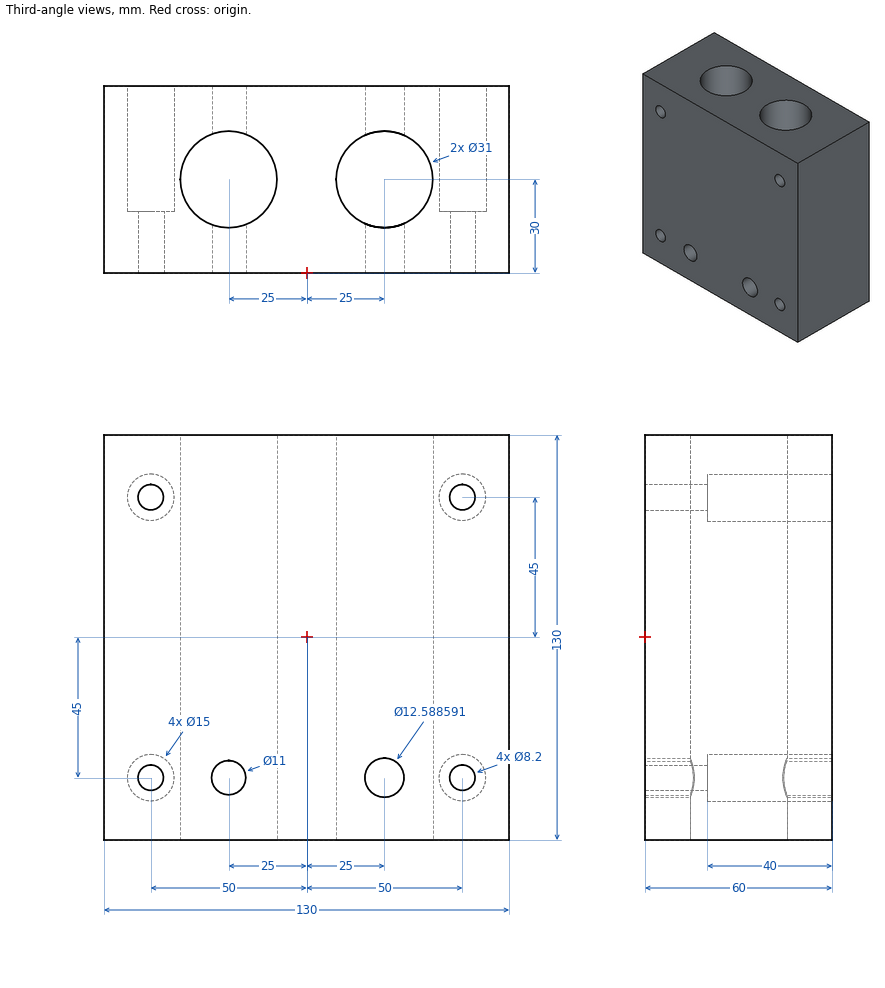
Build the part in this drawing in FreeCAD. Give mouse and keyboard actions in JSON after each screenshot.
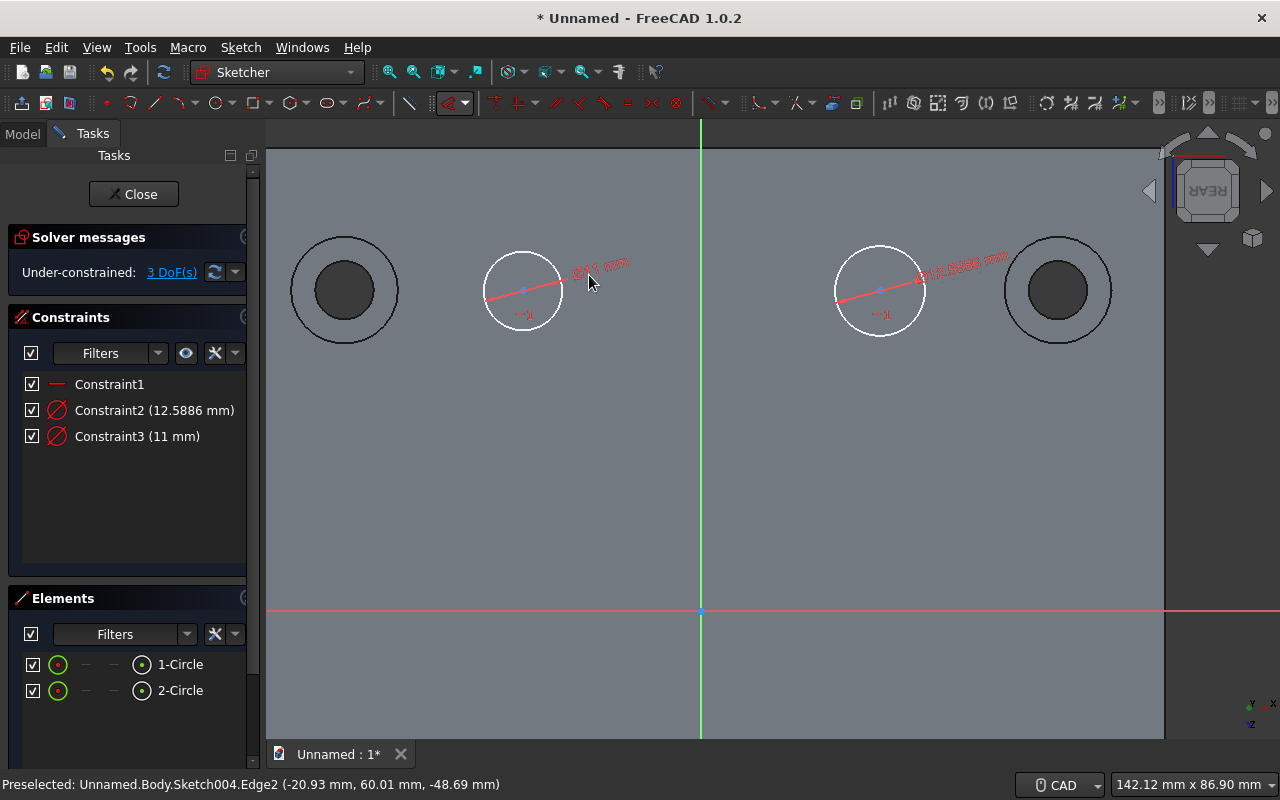
{"action": "left_click", "coordinate": [880, 291]}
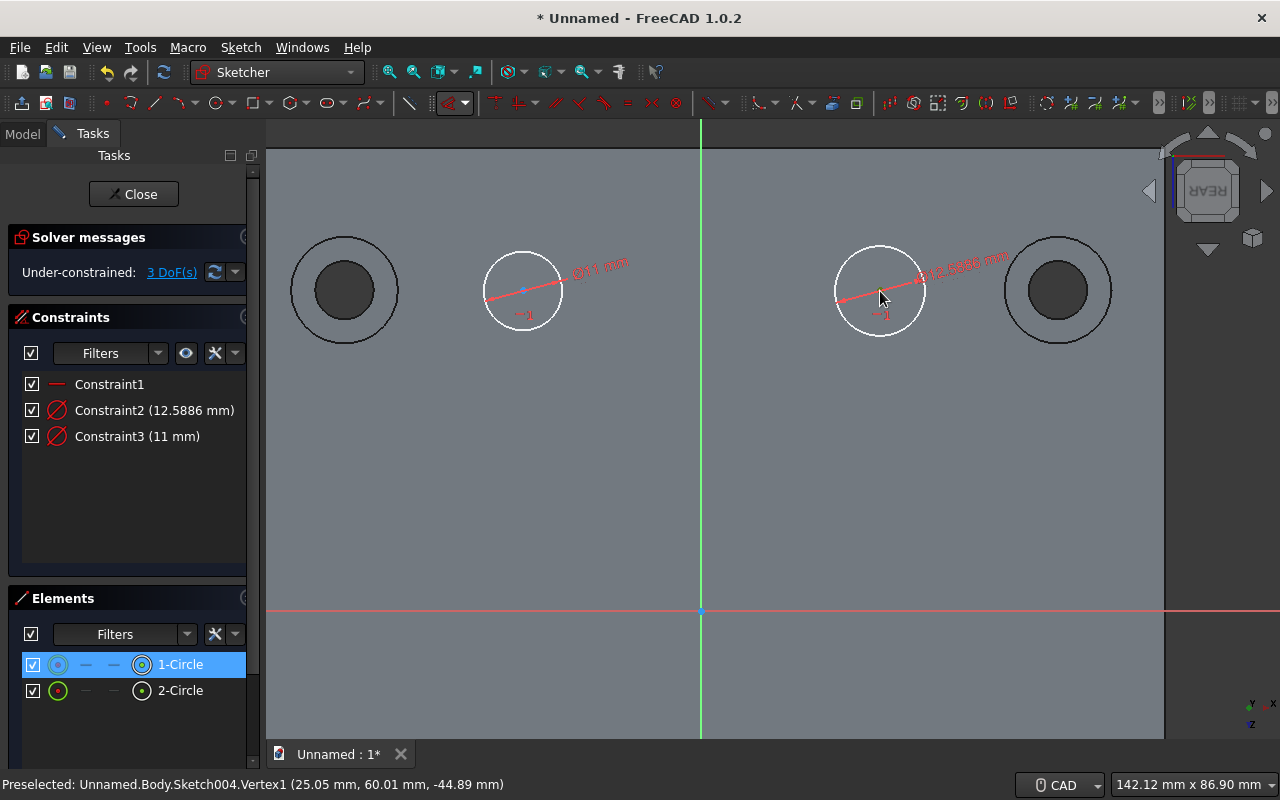
{"action": "key", "text": "l"}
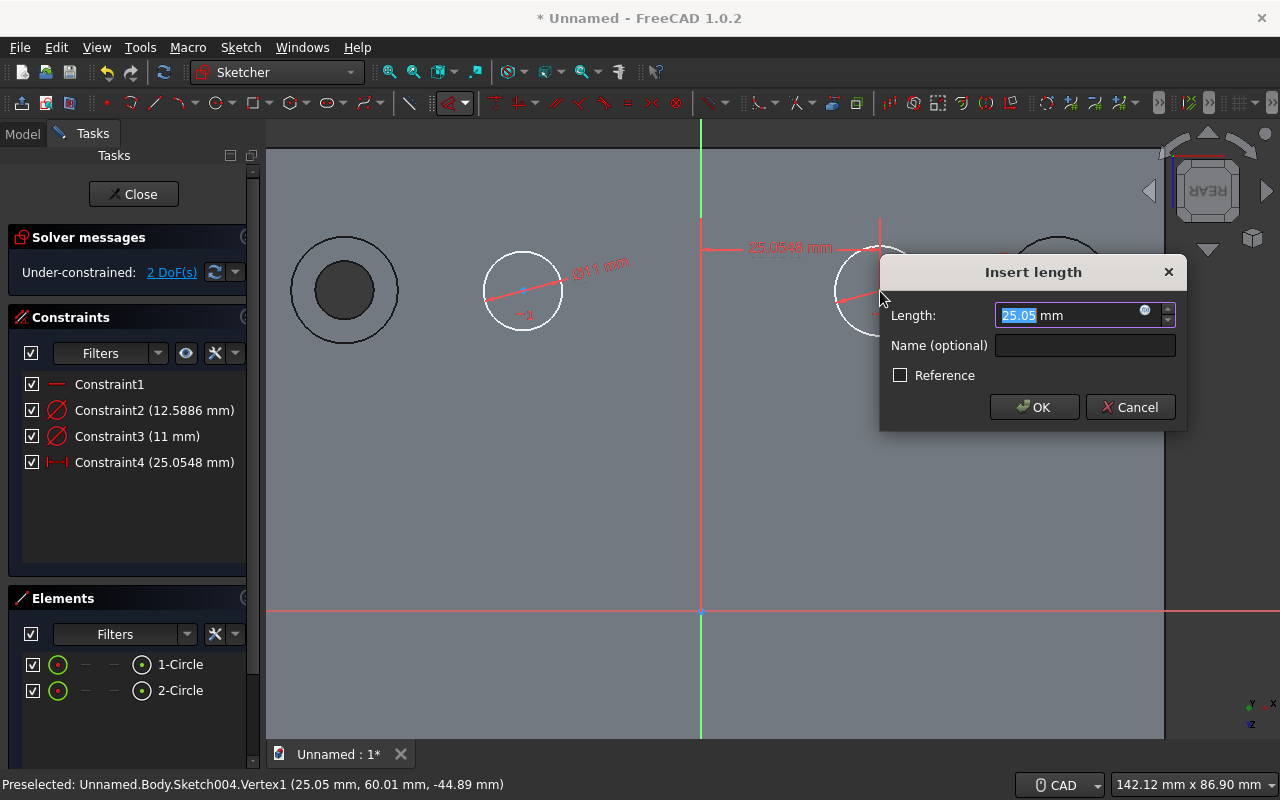
{"action": "type", "text": "25"}
{"action": "key", "text": "Return"}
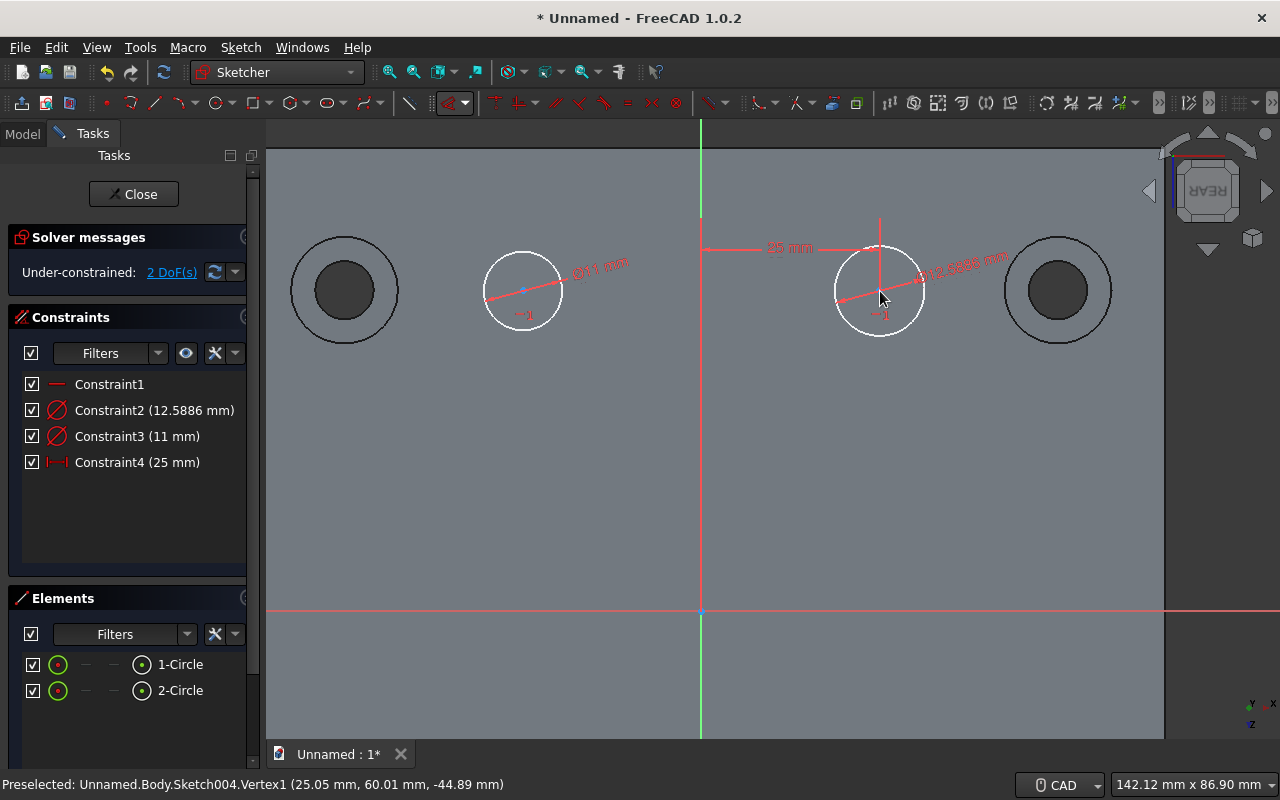
{"action": "left_click", "coordinate": [880, 291]}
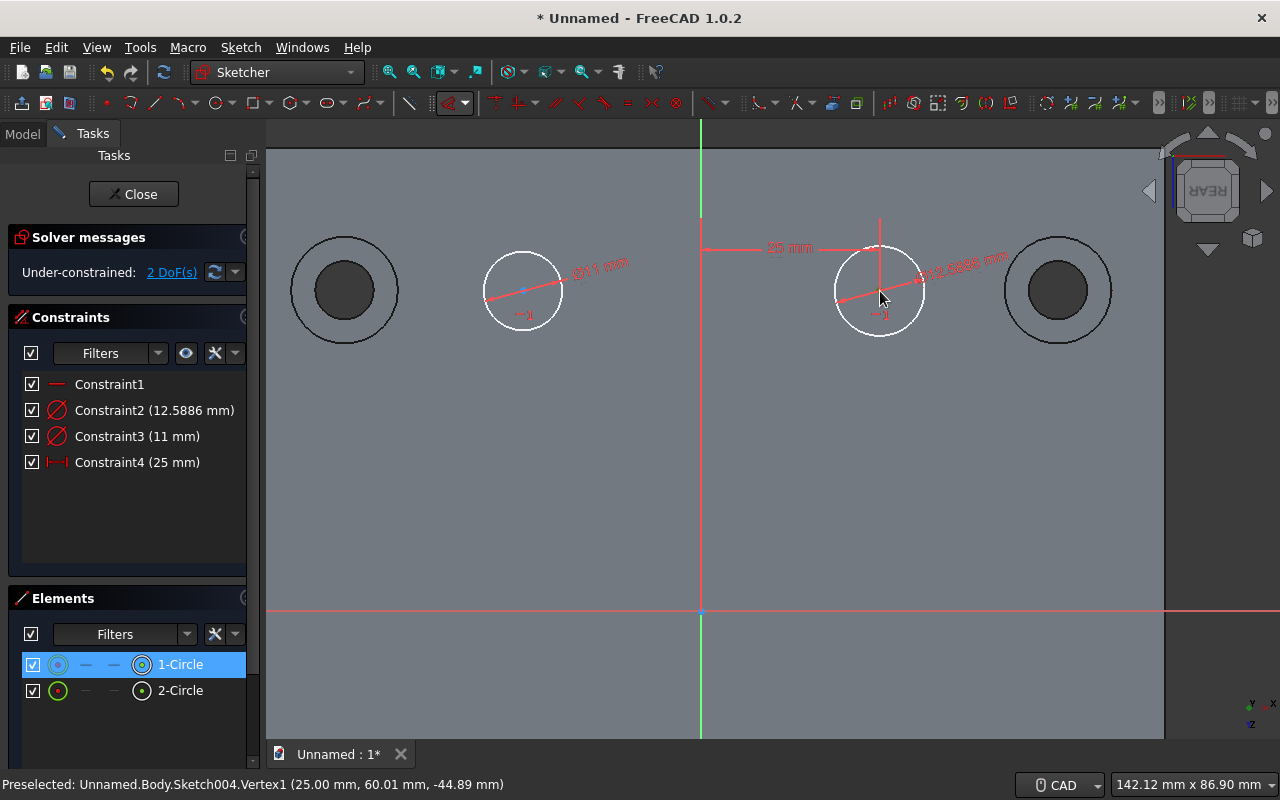
{"action": "key", "text": "i"}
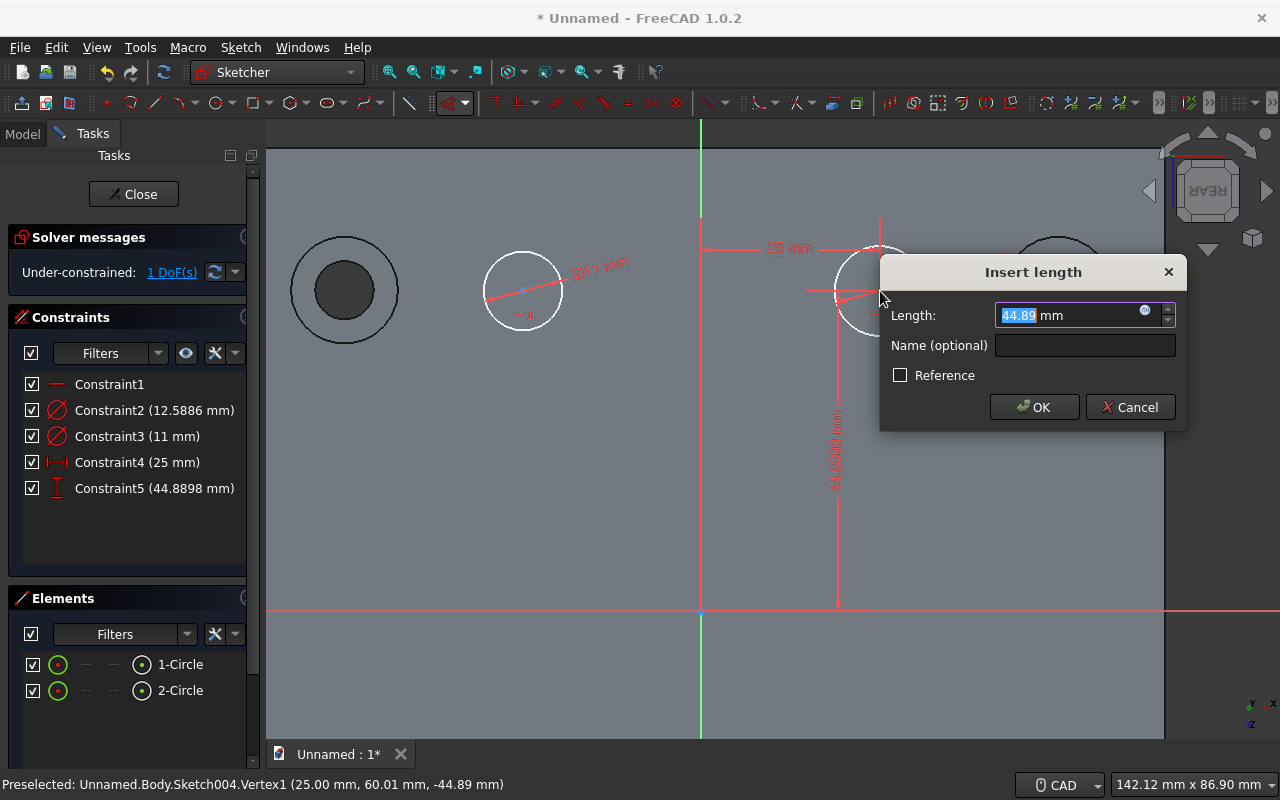
{"action": "type", "text": "45"}
{"action": "key", "text": "Return"}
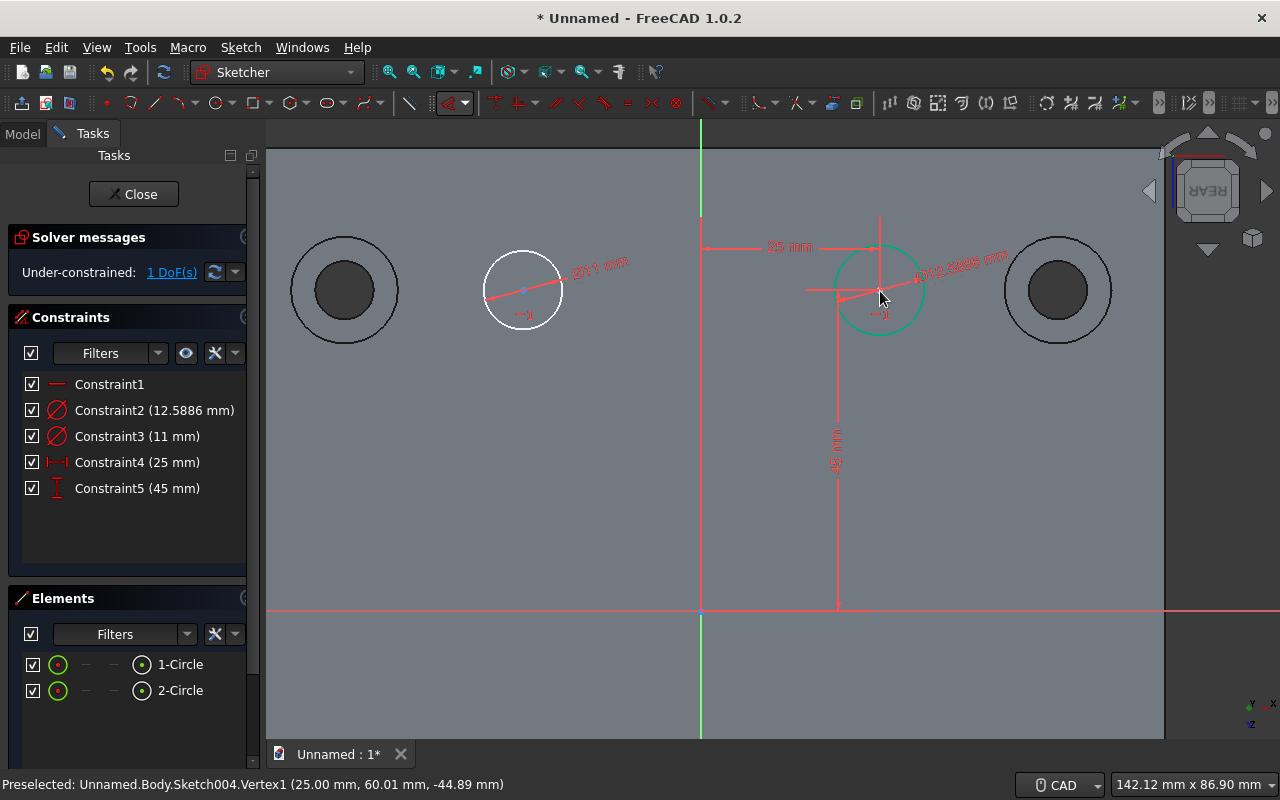
{"action": "left_click", "coordinate": [523, 290]}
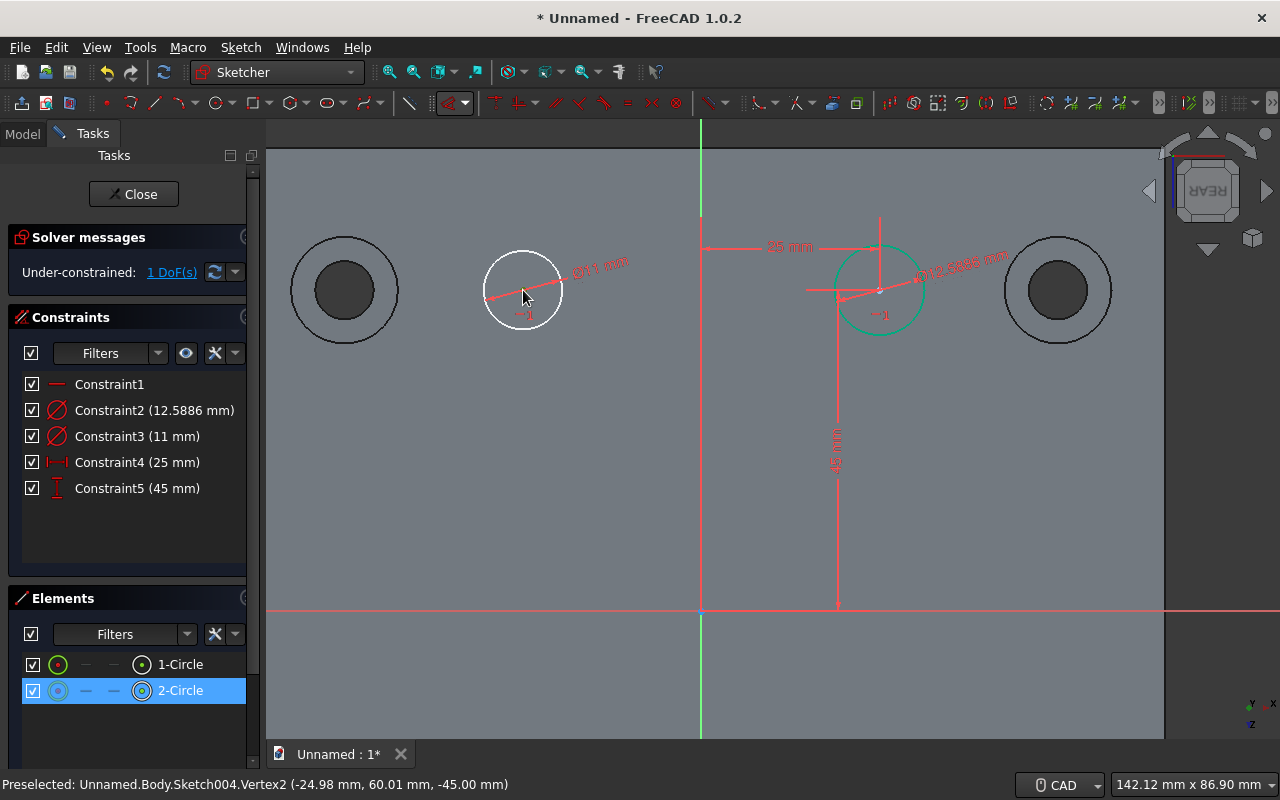
{"action": "left_click", "coordinate": [468, 104]}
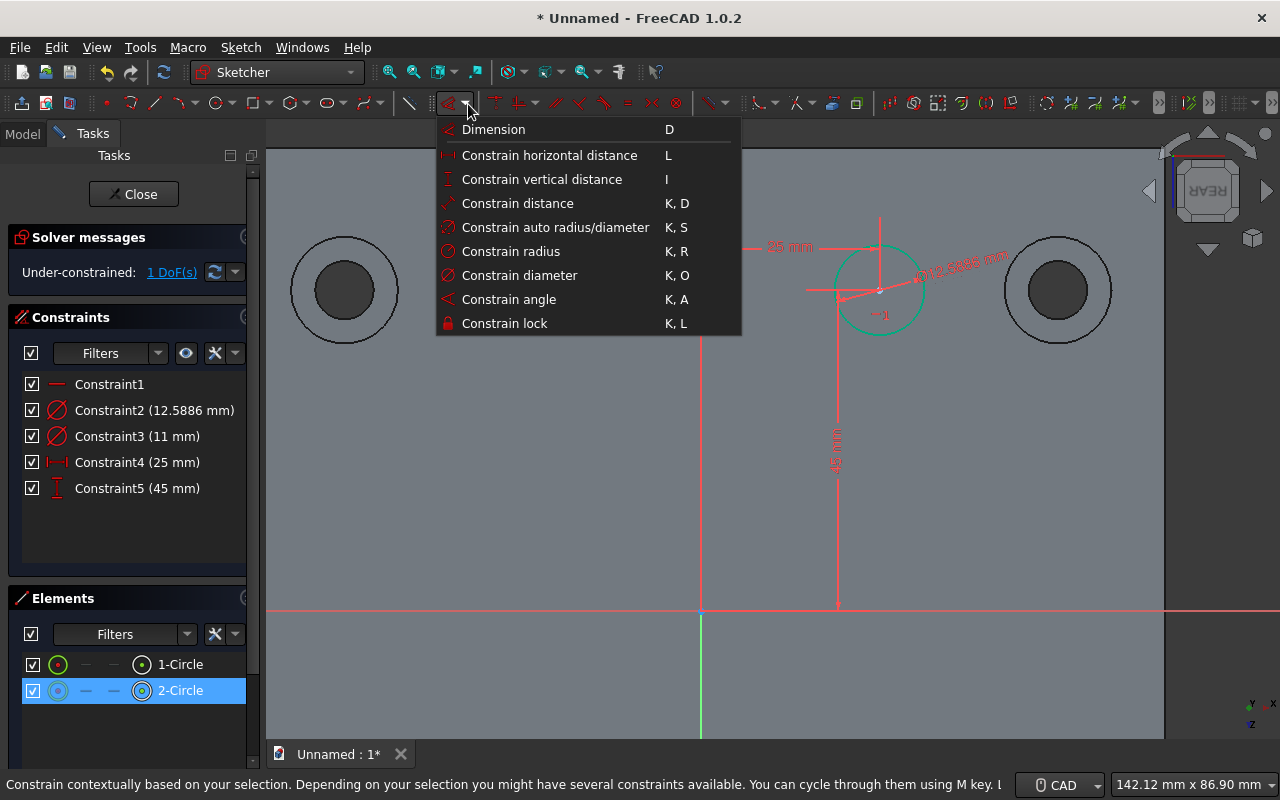
{"action": "left_click", "coordinate": [589, 155]}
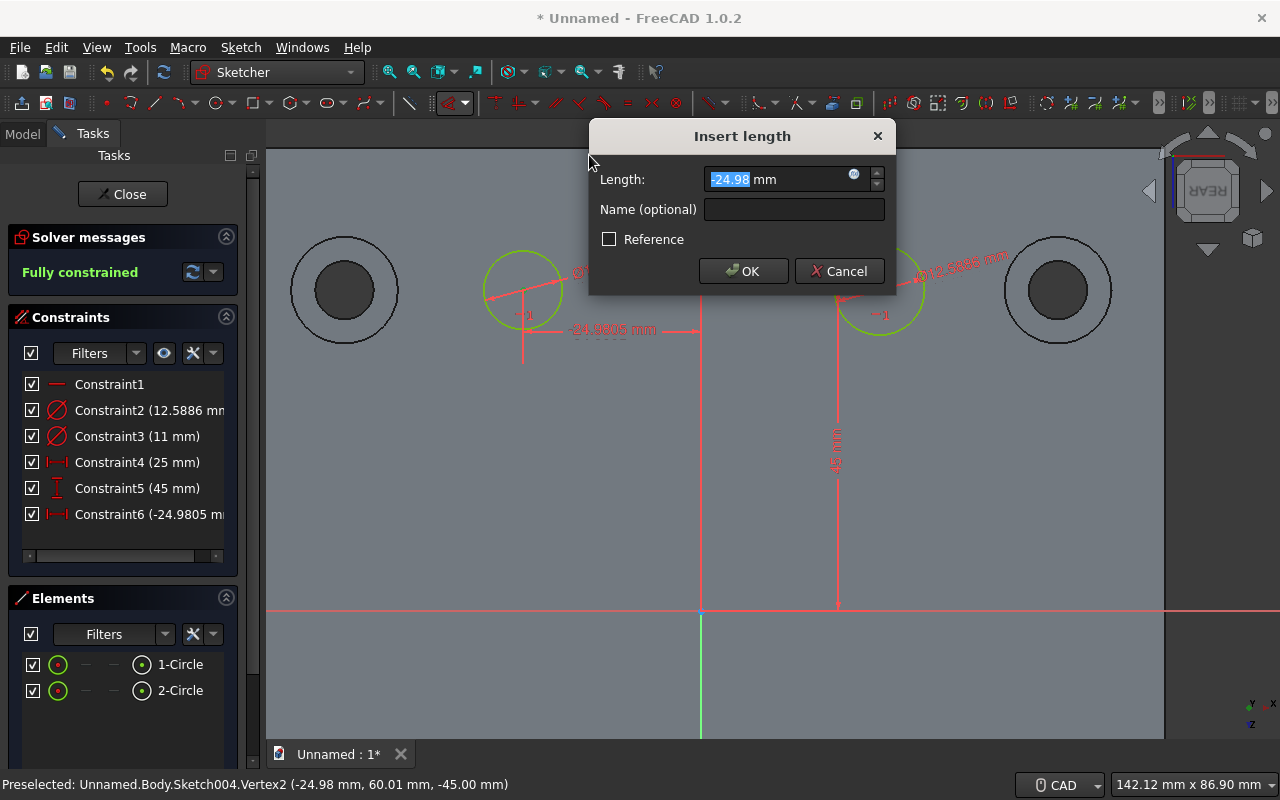
{"action": "type", "text": "-25"}
{"action": "key", "text": "Return"}